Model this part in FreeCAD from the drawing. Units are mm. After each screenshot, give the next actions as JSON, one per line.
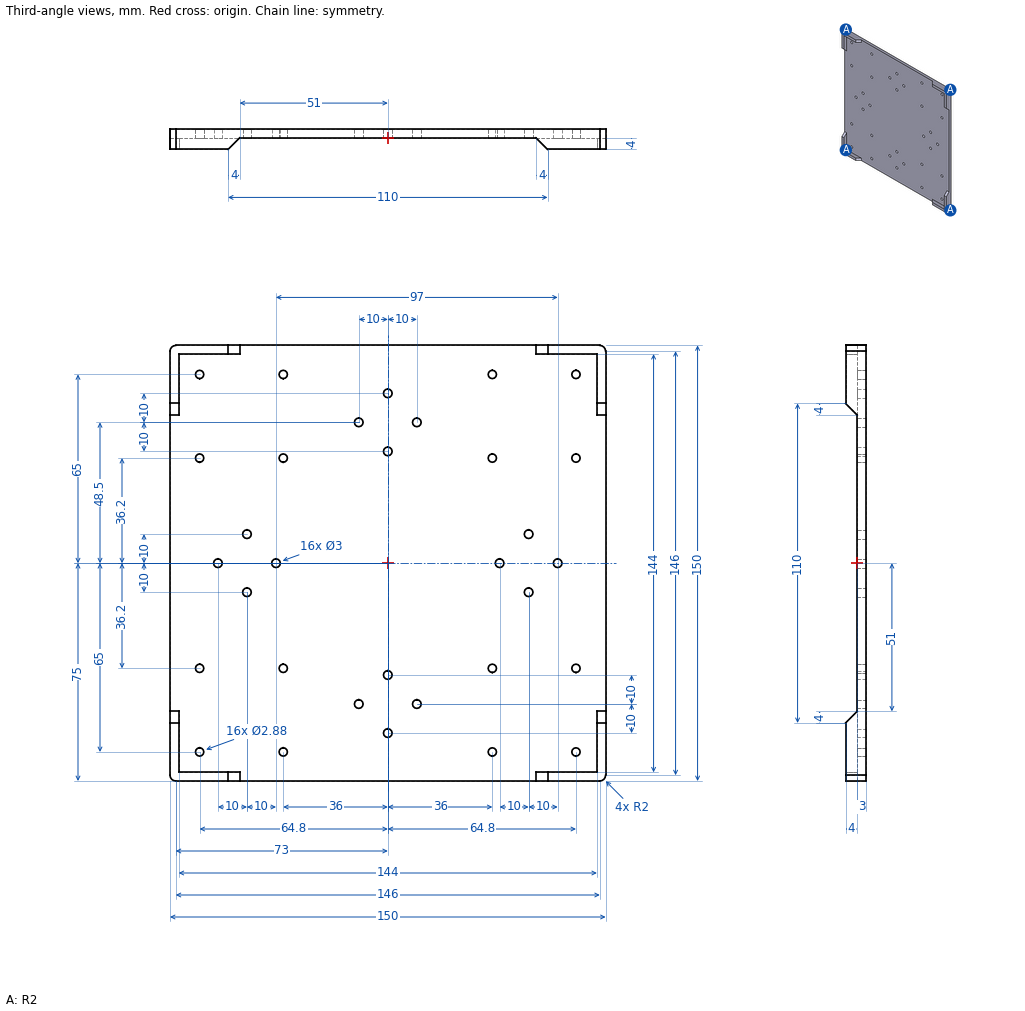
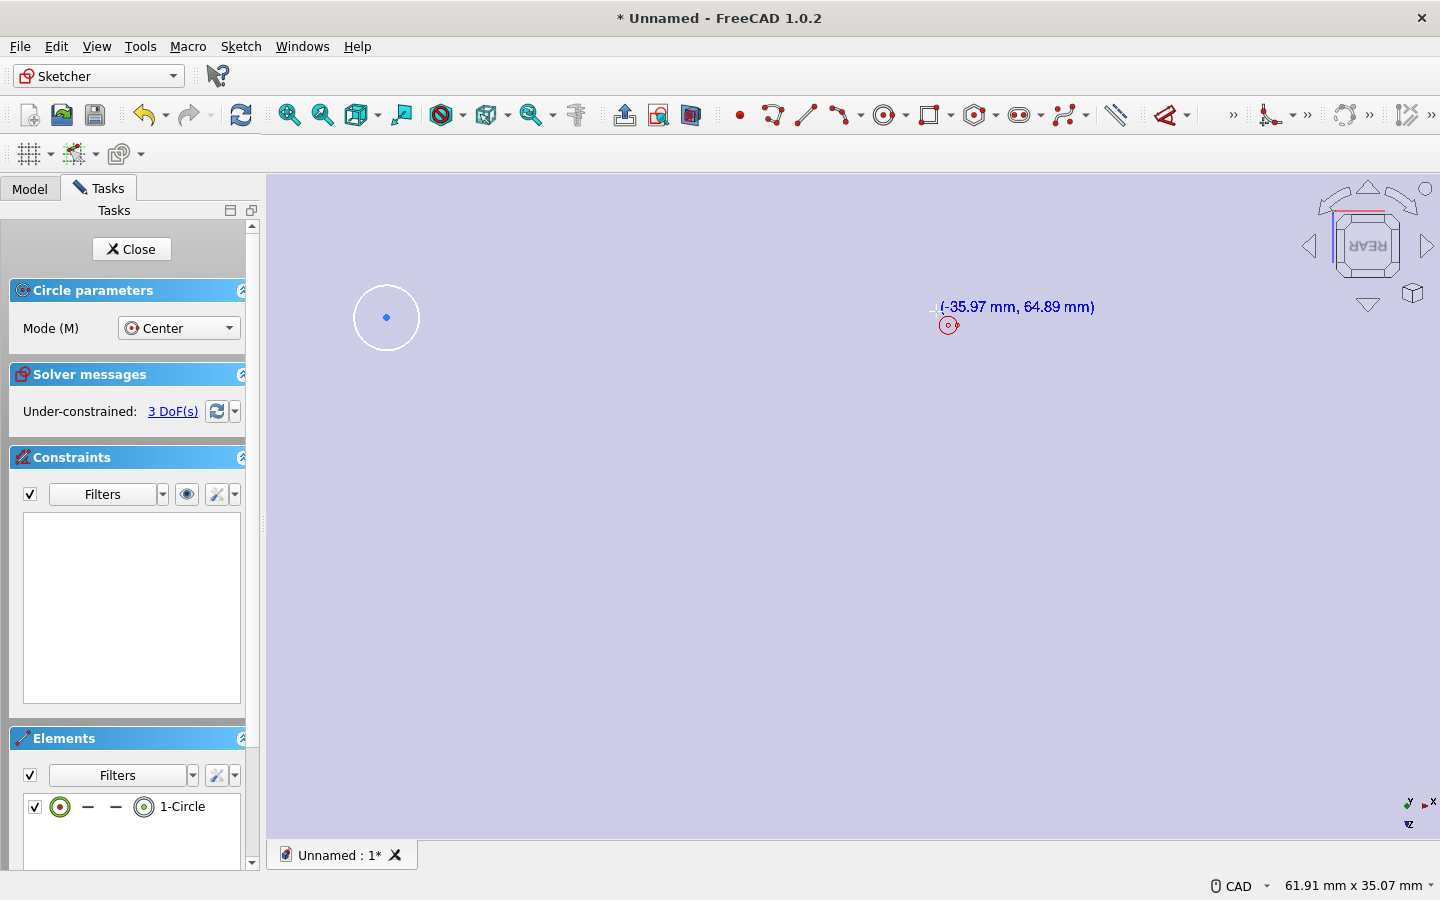
{"action": "scroll", "coordinate": [619, 301], "scroll_direction": "down", "scroll_amount": 9}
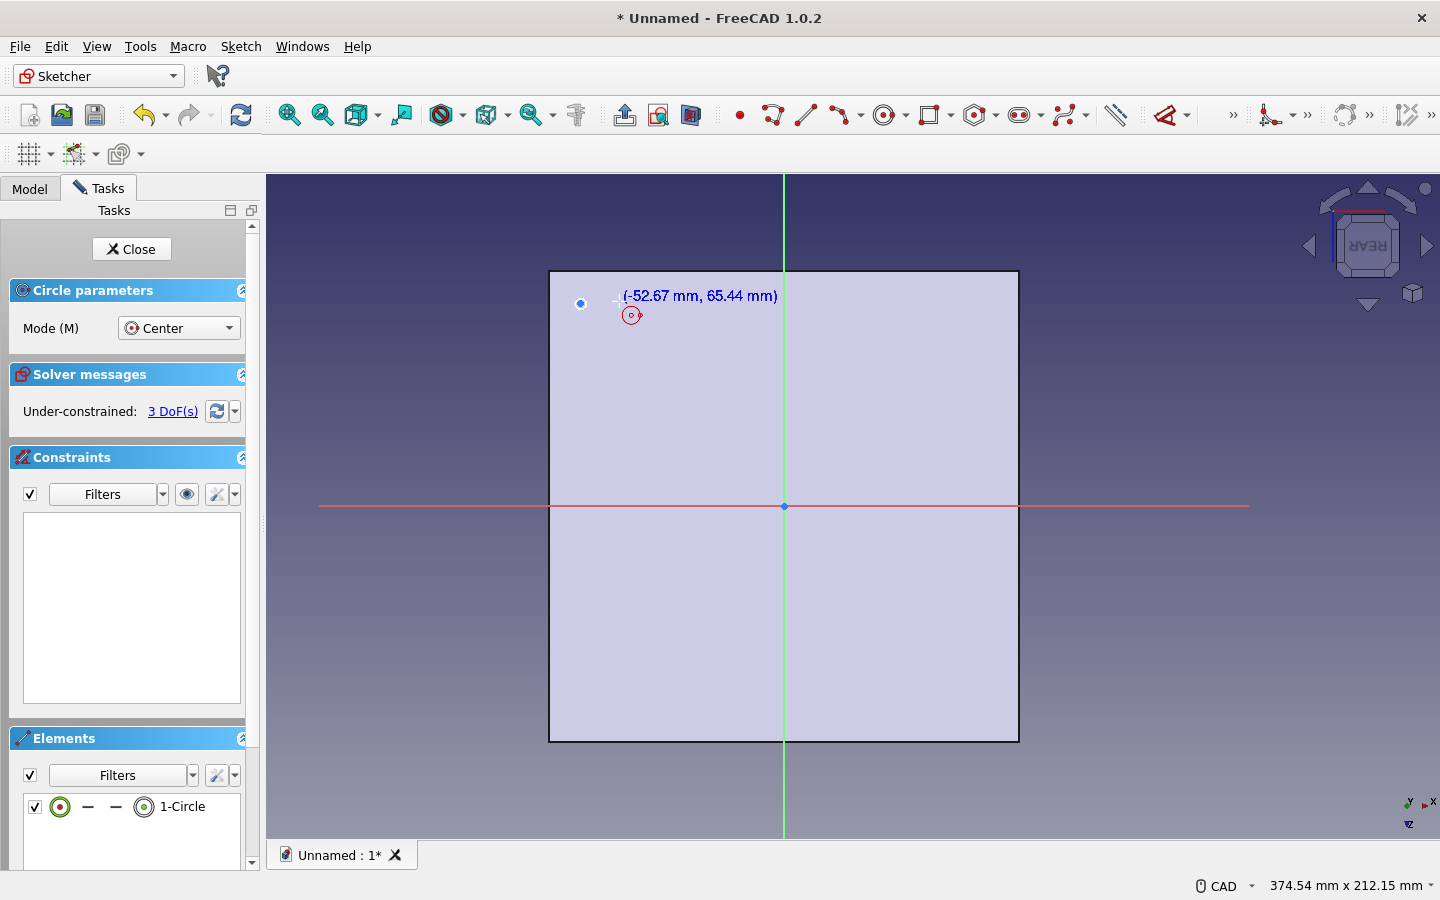
{"action": "left_click", "coordinate": [671, 303]}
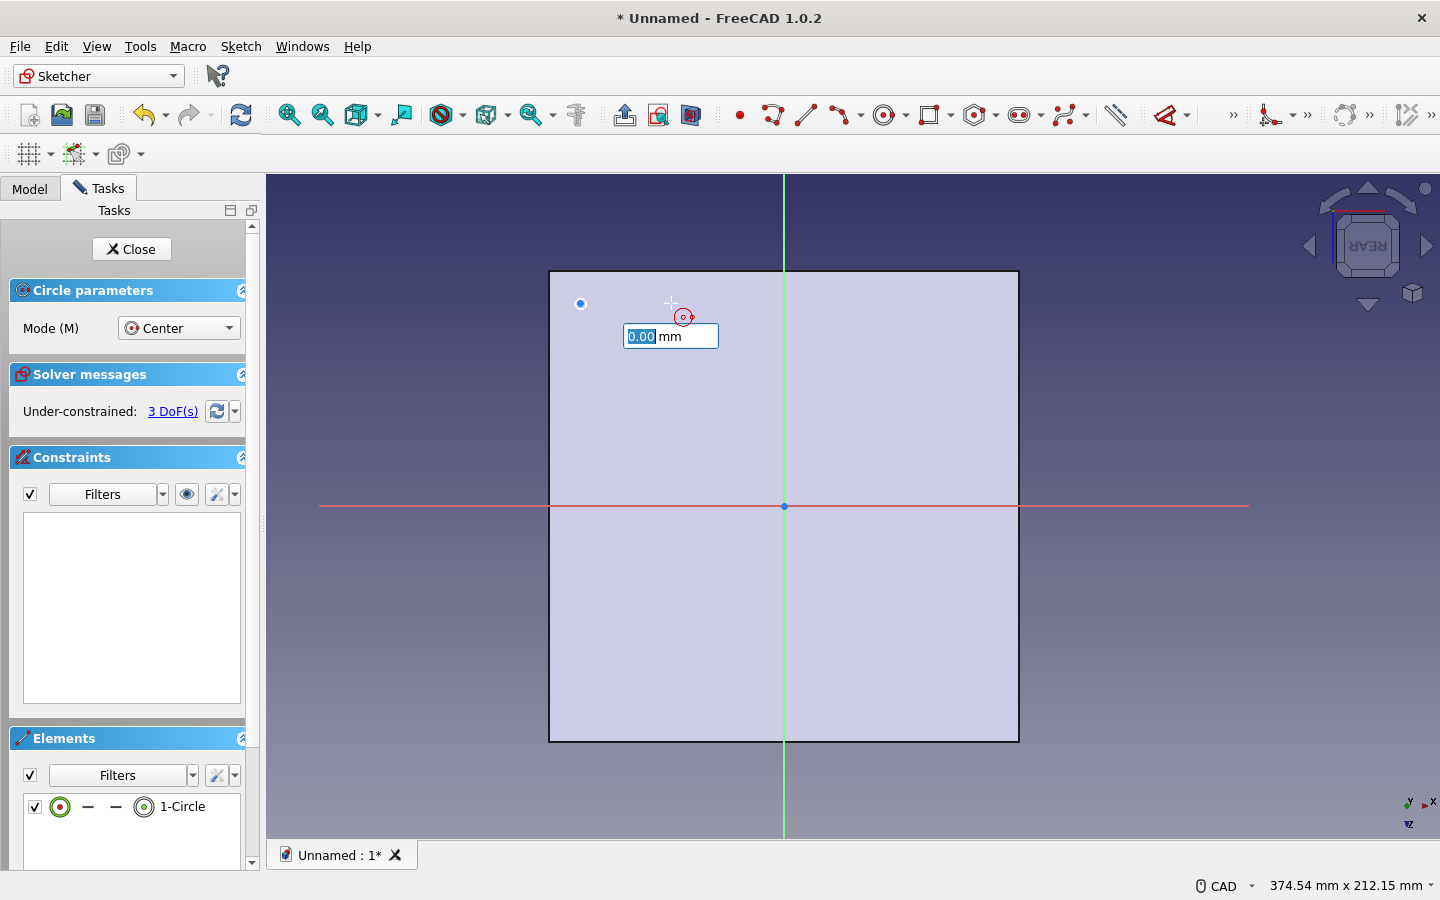
{"action": "scroll", "coordinate": [675, 300], "scroll_direction": "up", "scroll_amount": 7}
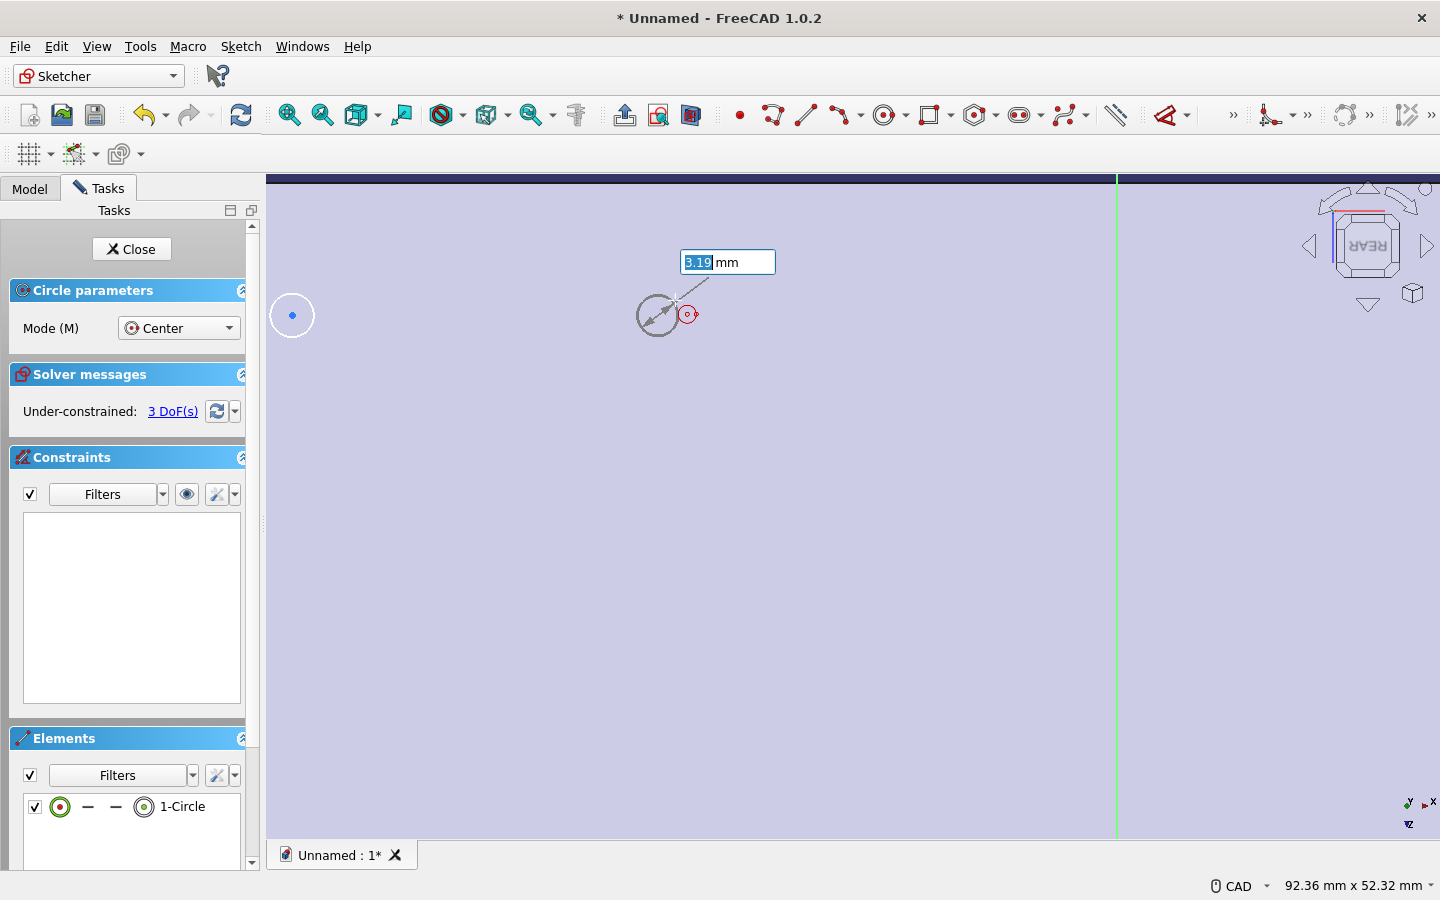
{"action": "left_click", "coordinate": [673, 297]}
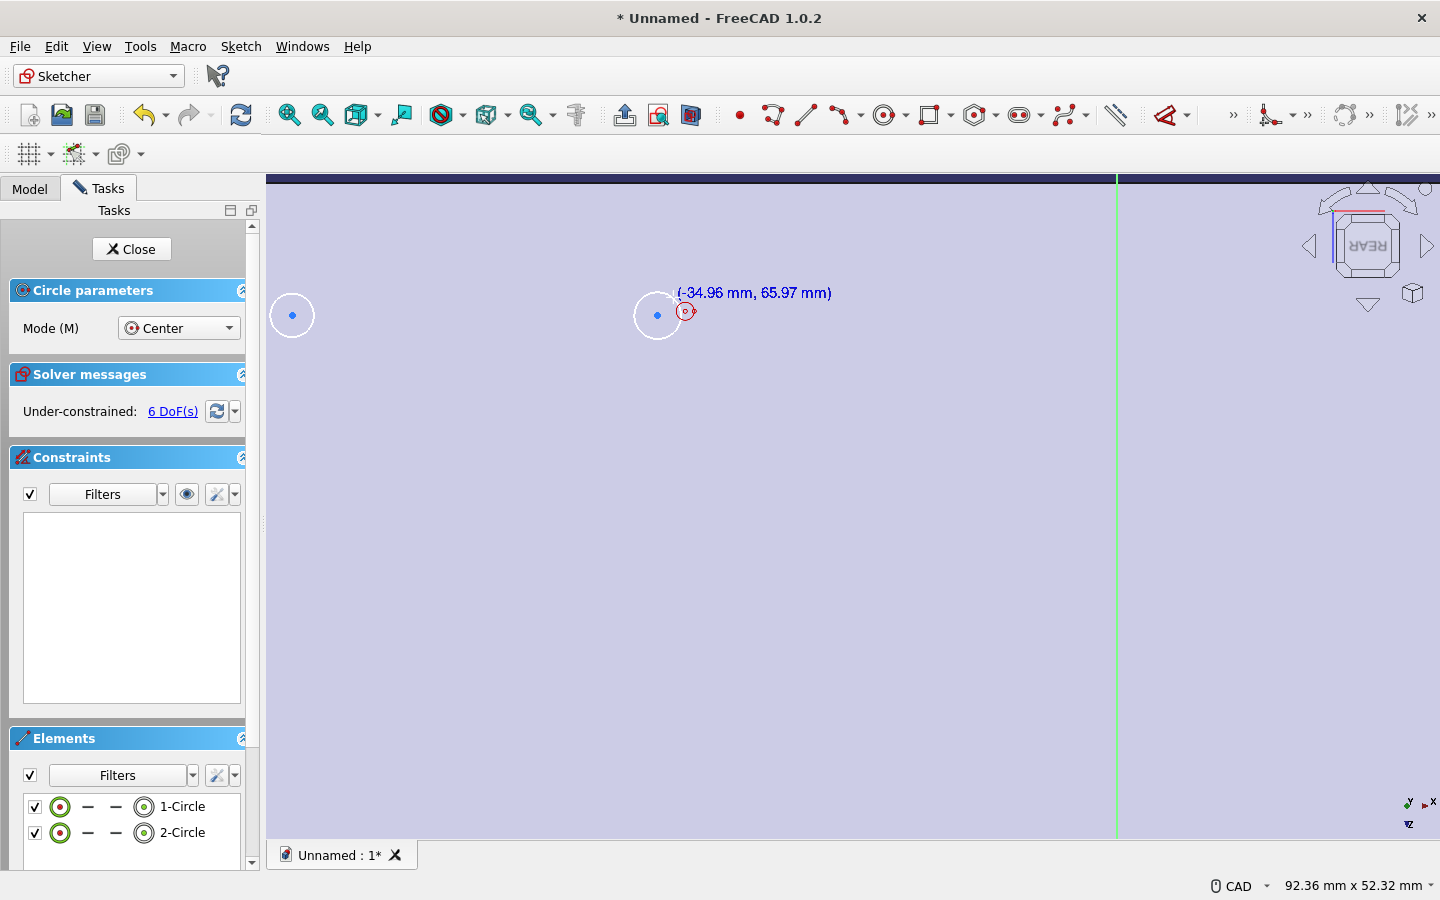
{"action": "scroll", "coordinate": [676, 300], "scroll_direction": "down", "scroll_amount": 7}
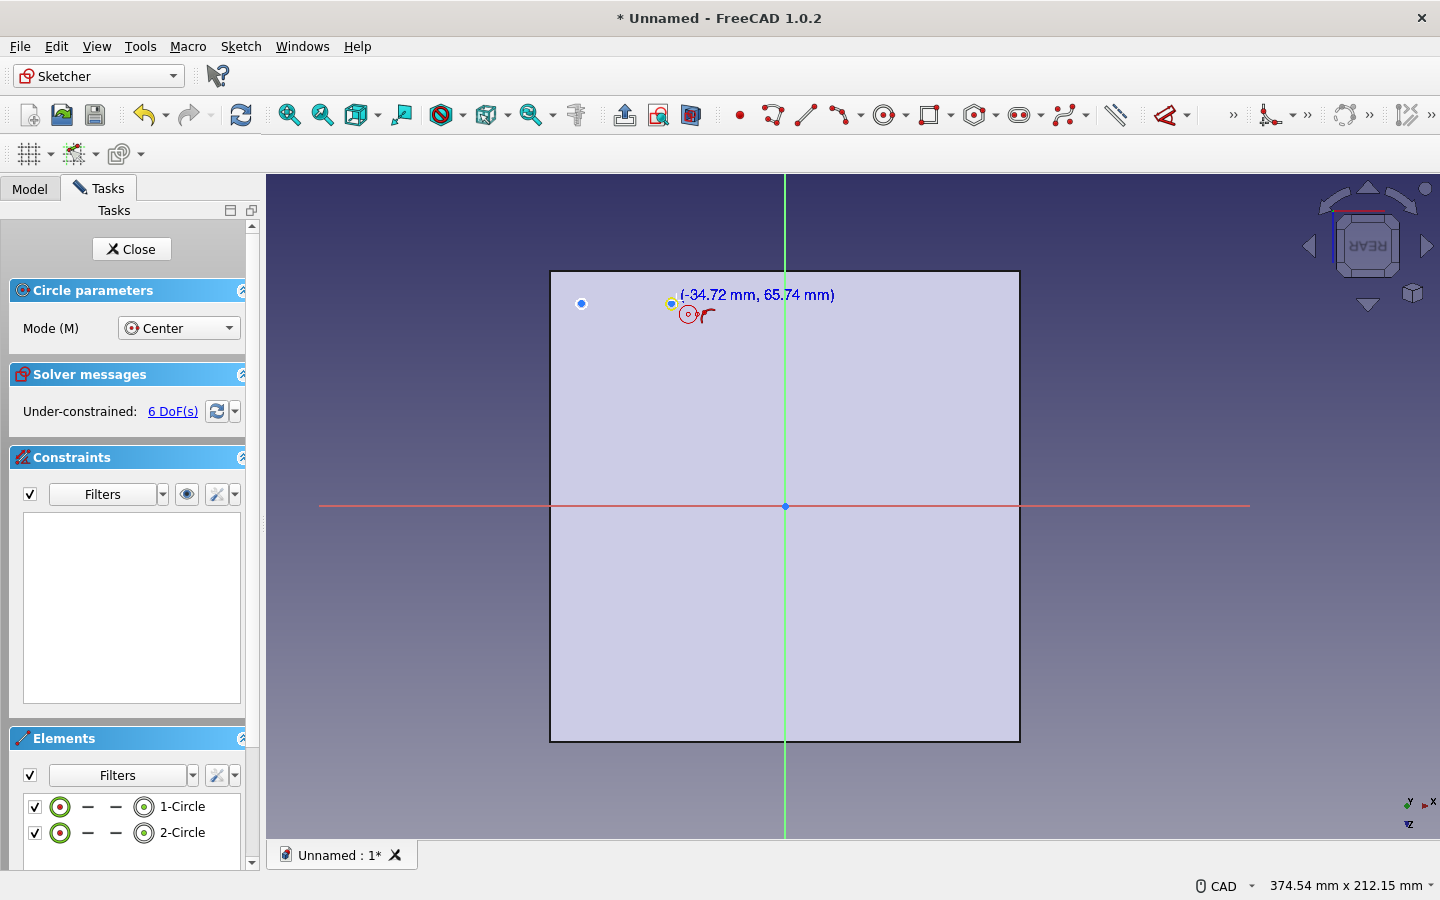
{"action": "scroll", "coordinate": [582, 393], "scroll_direction": "up", "scroll_amount": 9}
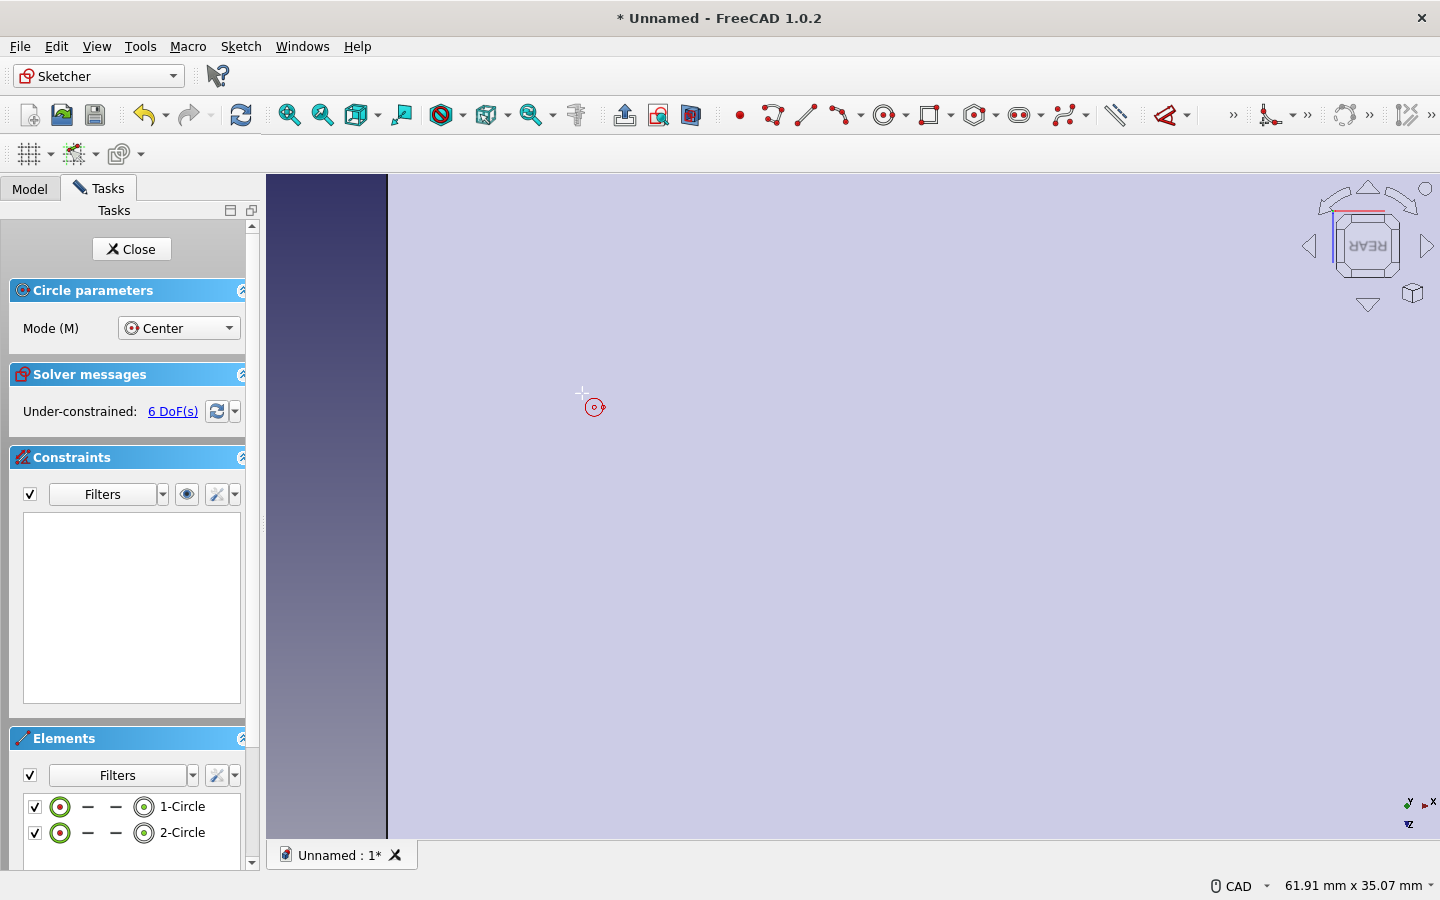
{"action": "scroll", "coordinate": [582, 393], "scroll_direction": "down", "scroll_amount": 9}